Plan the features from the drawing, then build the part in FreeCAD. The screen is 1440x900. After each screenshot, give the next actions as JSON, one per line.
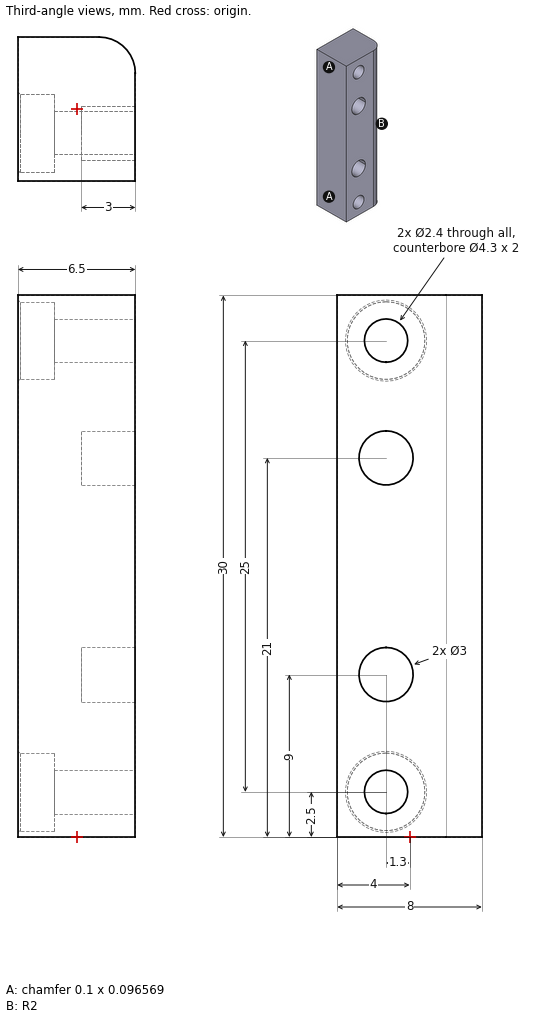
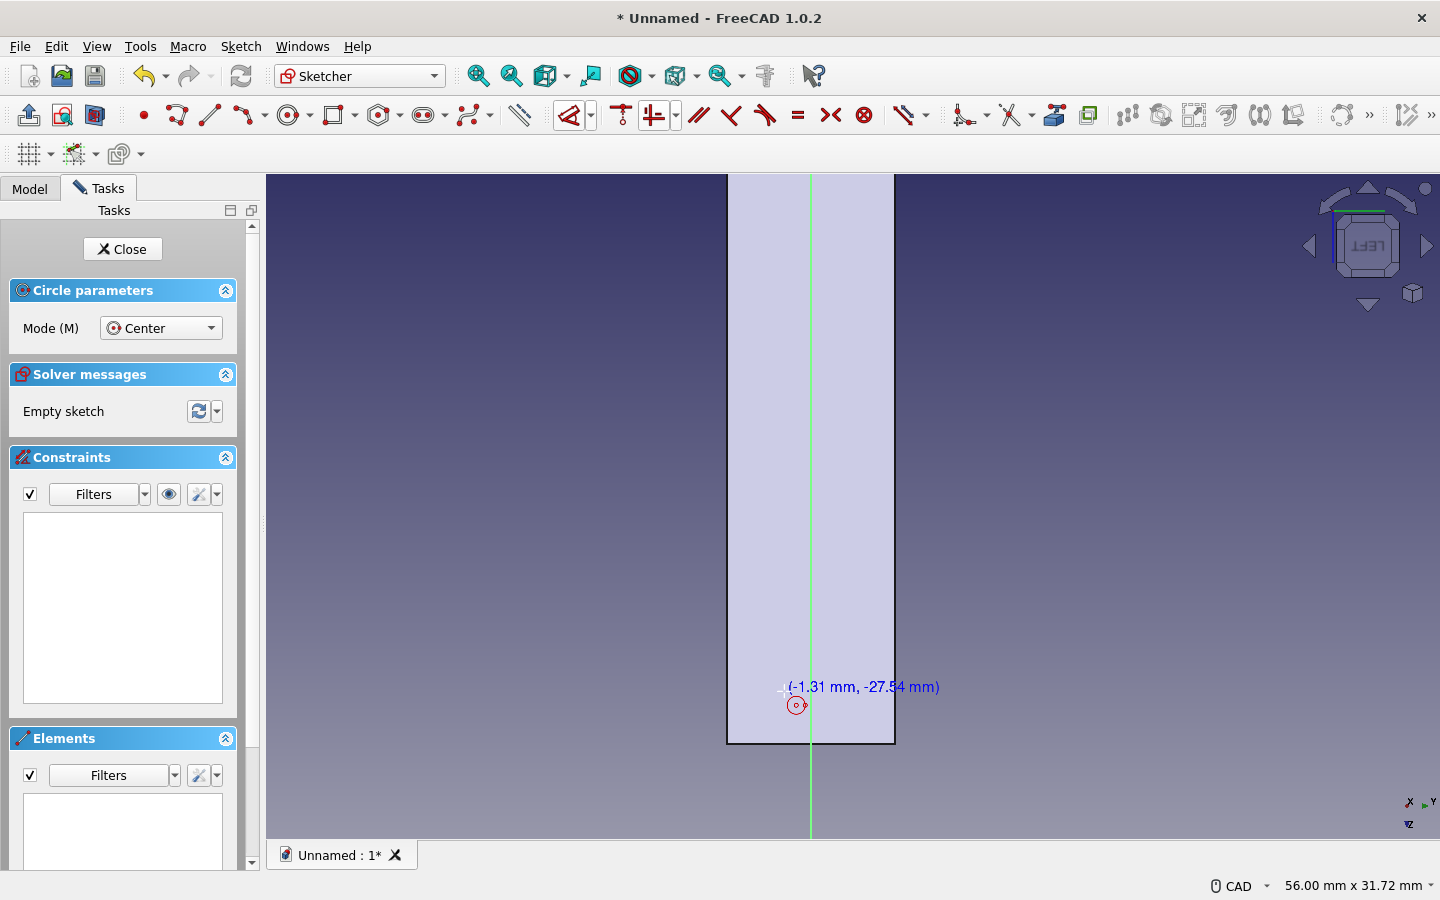
{"action": "left_click", "coordinate": [784, 691]}
{"action": "mouse_move", "coordinate": [766, 673]}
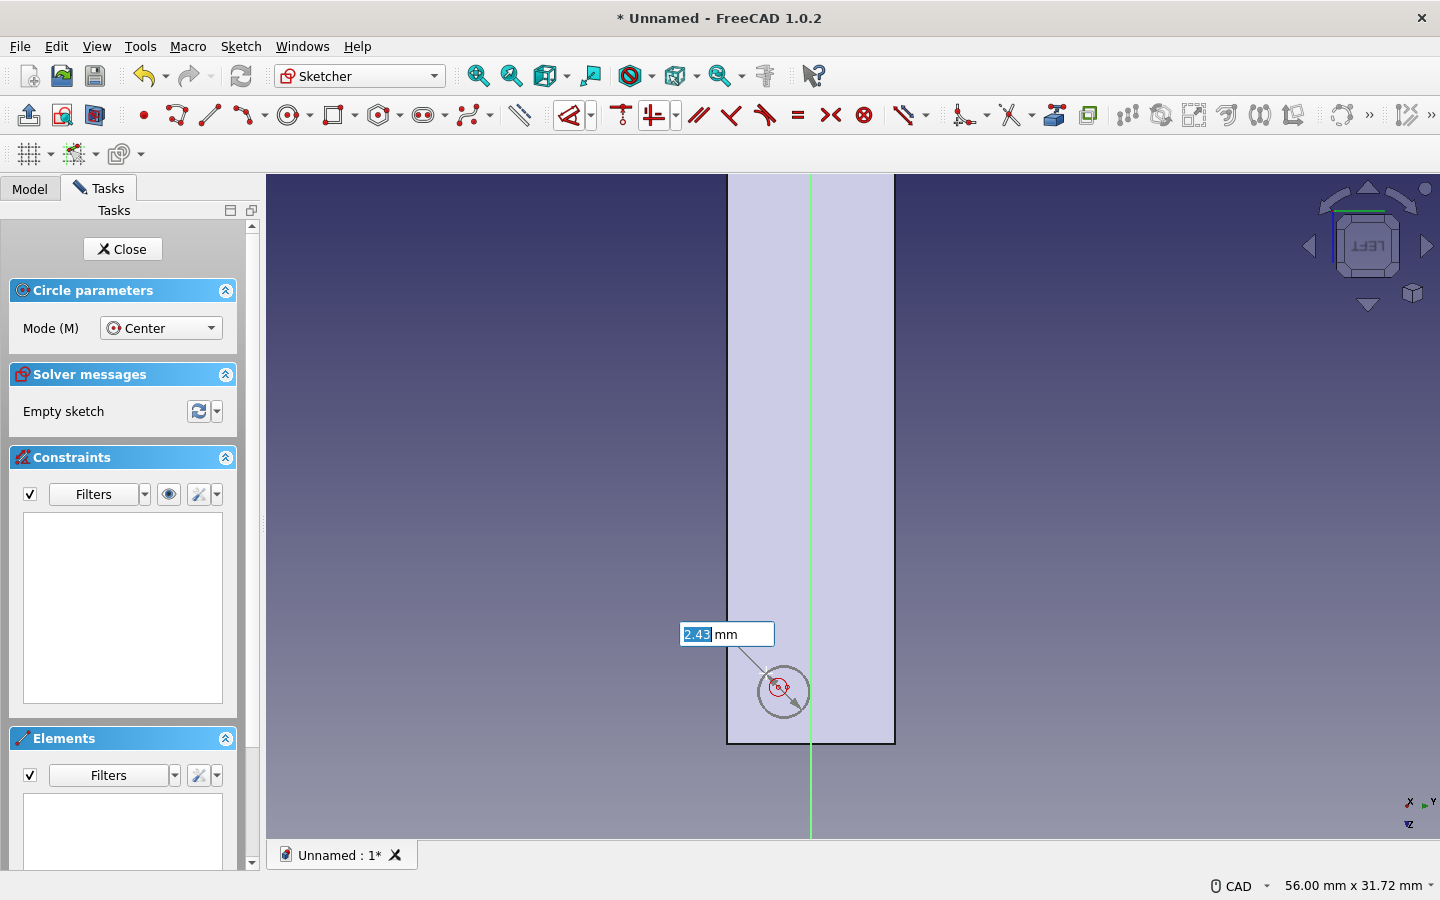
{"action": "type", "text": "2.4"}
{"action": "key", "text": "Return"}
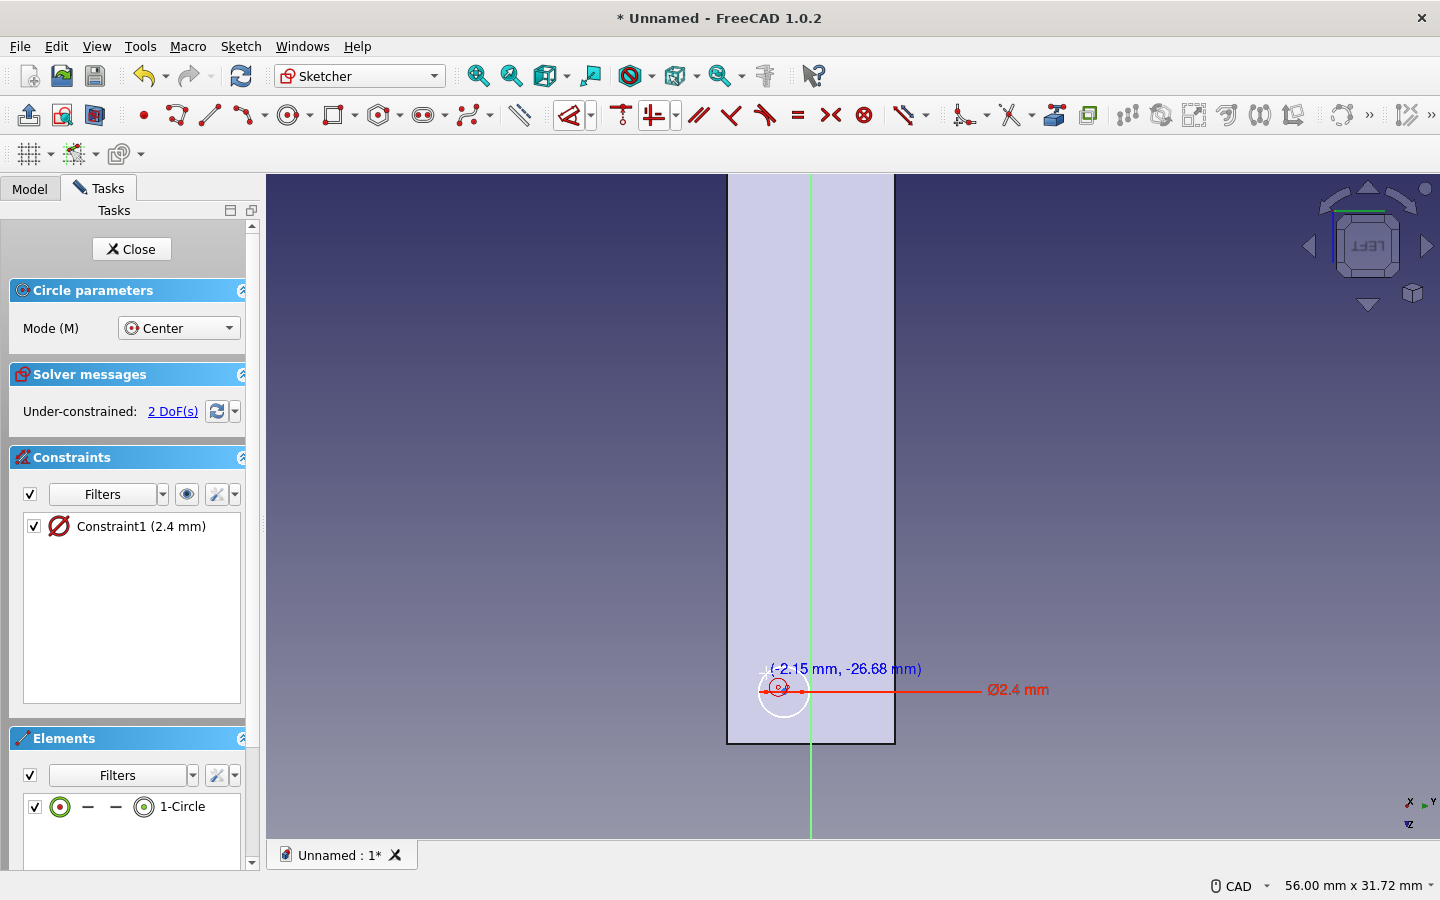
{"action": "scroll", "coordinate": [784, 691], "scroll_direction": "down", "scroll_amount": 2}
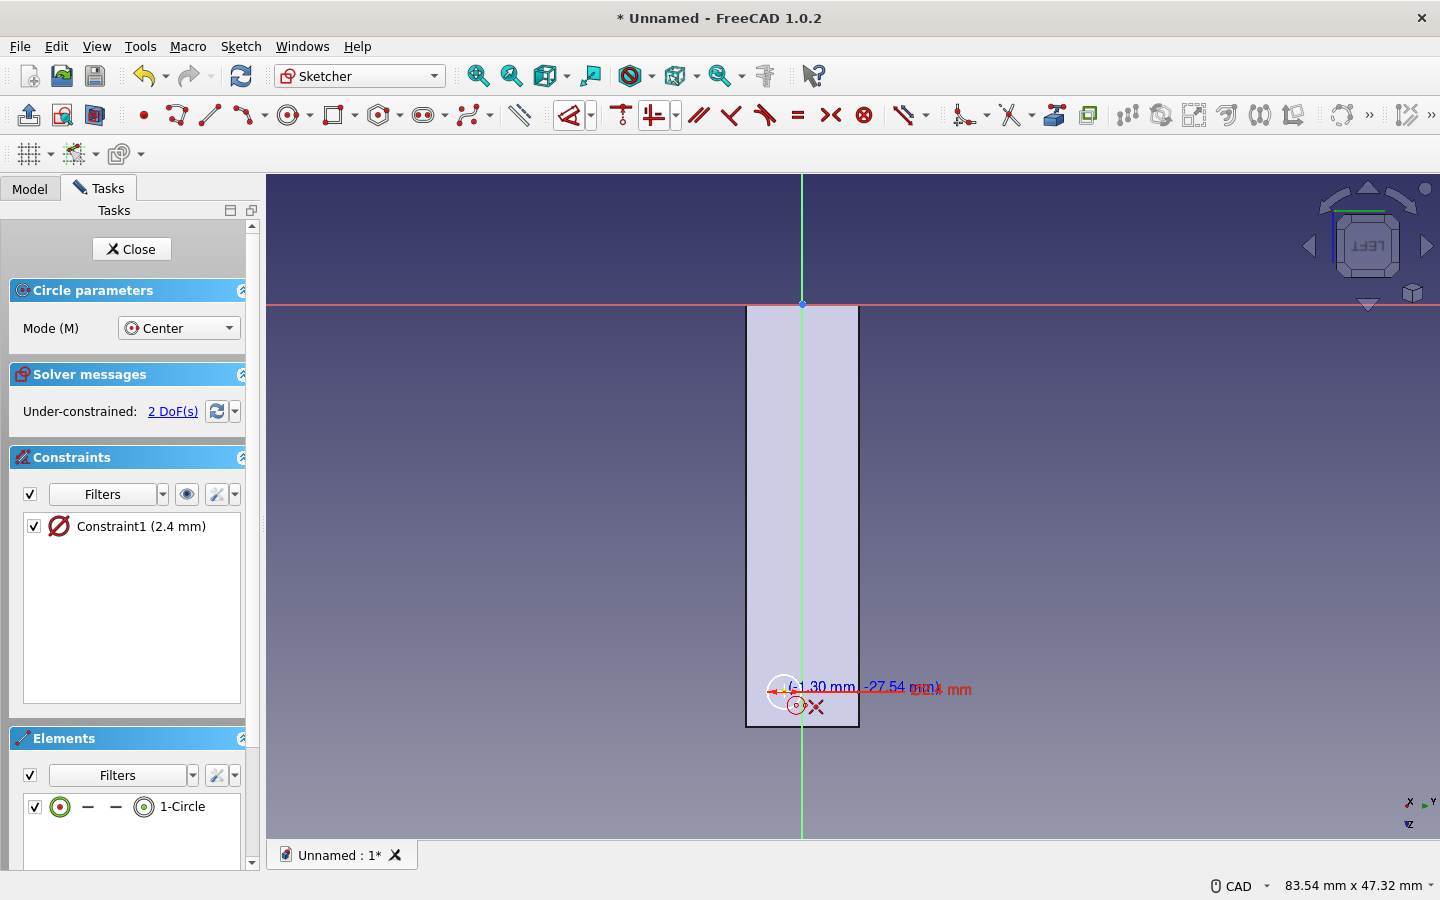
{"action": "scroll", "coordinate": [784, 340], "scroll_direction": "up", "scroll_amount": 2}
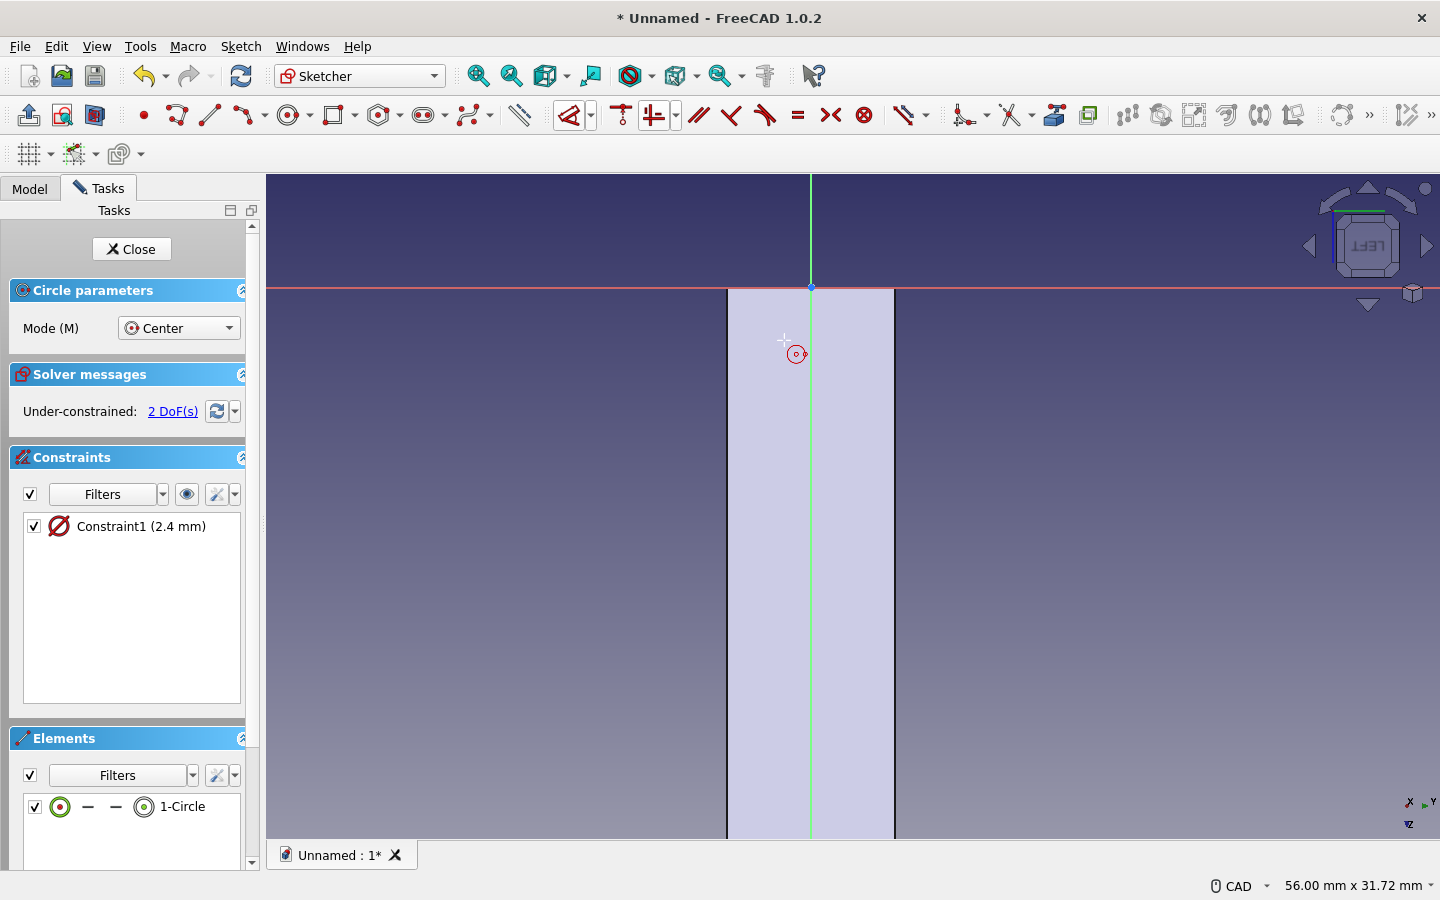
{"action": "left_click", "coordinate": [784, 340]}
{"action": "mouse_move", "coordinate": [766, 322]}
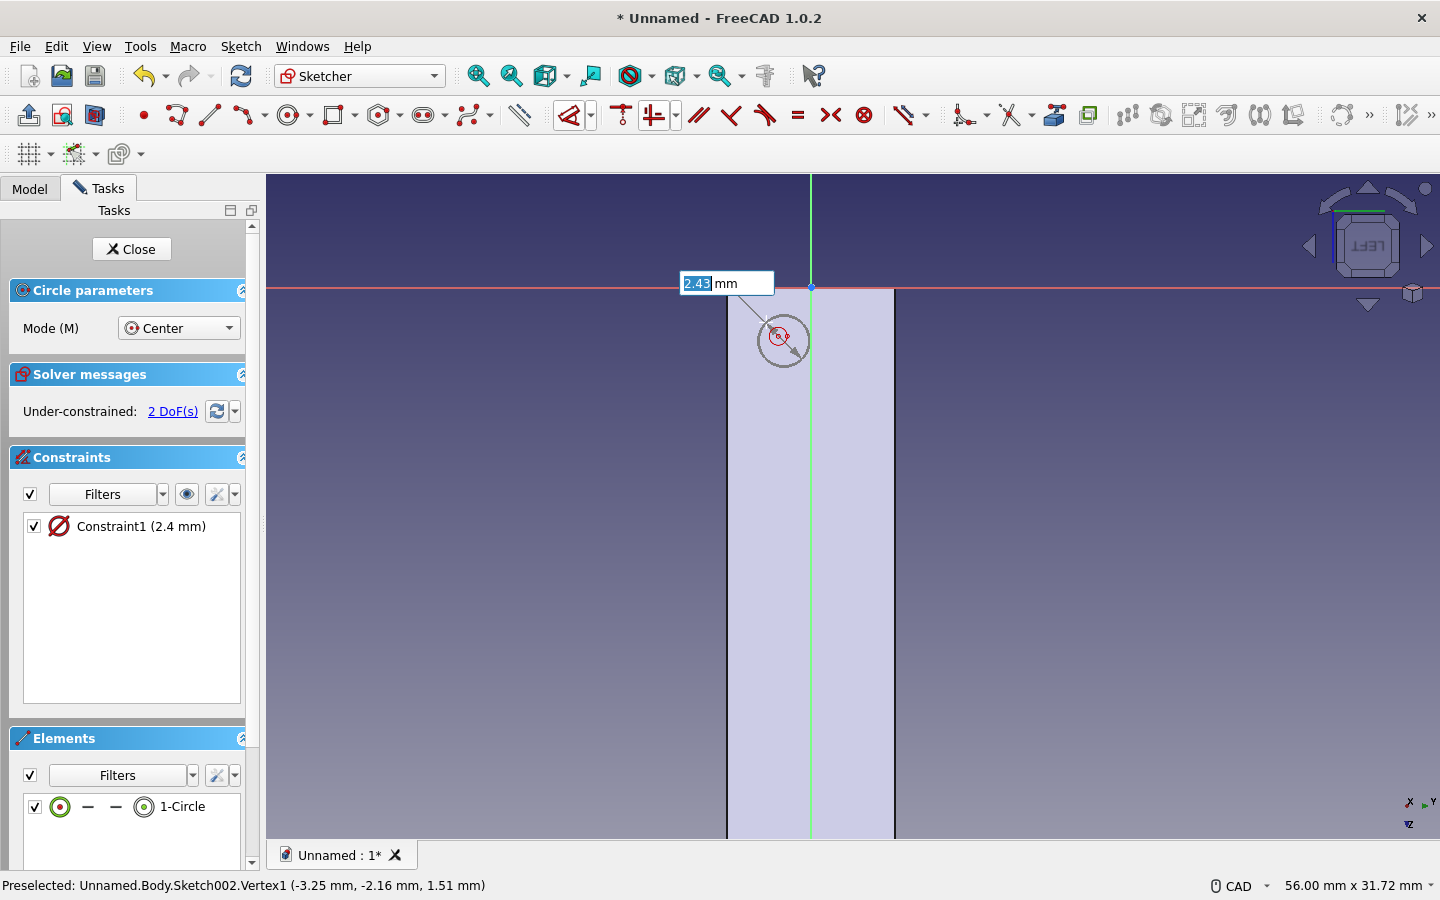
{"action": "type", "text": "2.4"}
{"action": "key", "text": "Return"}
{"action": "key", "text": "Escape"}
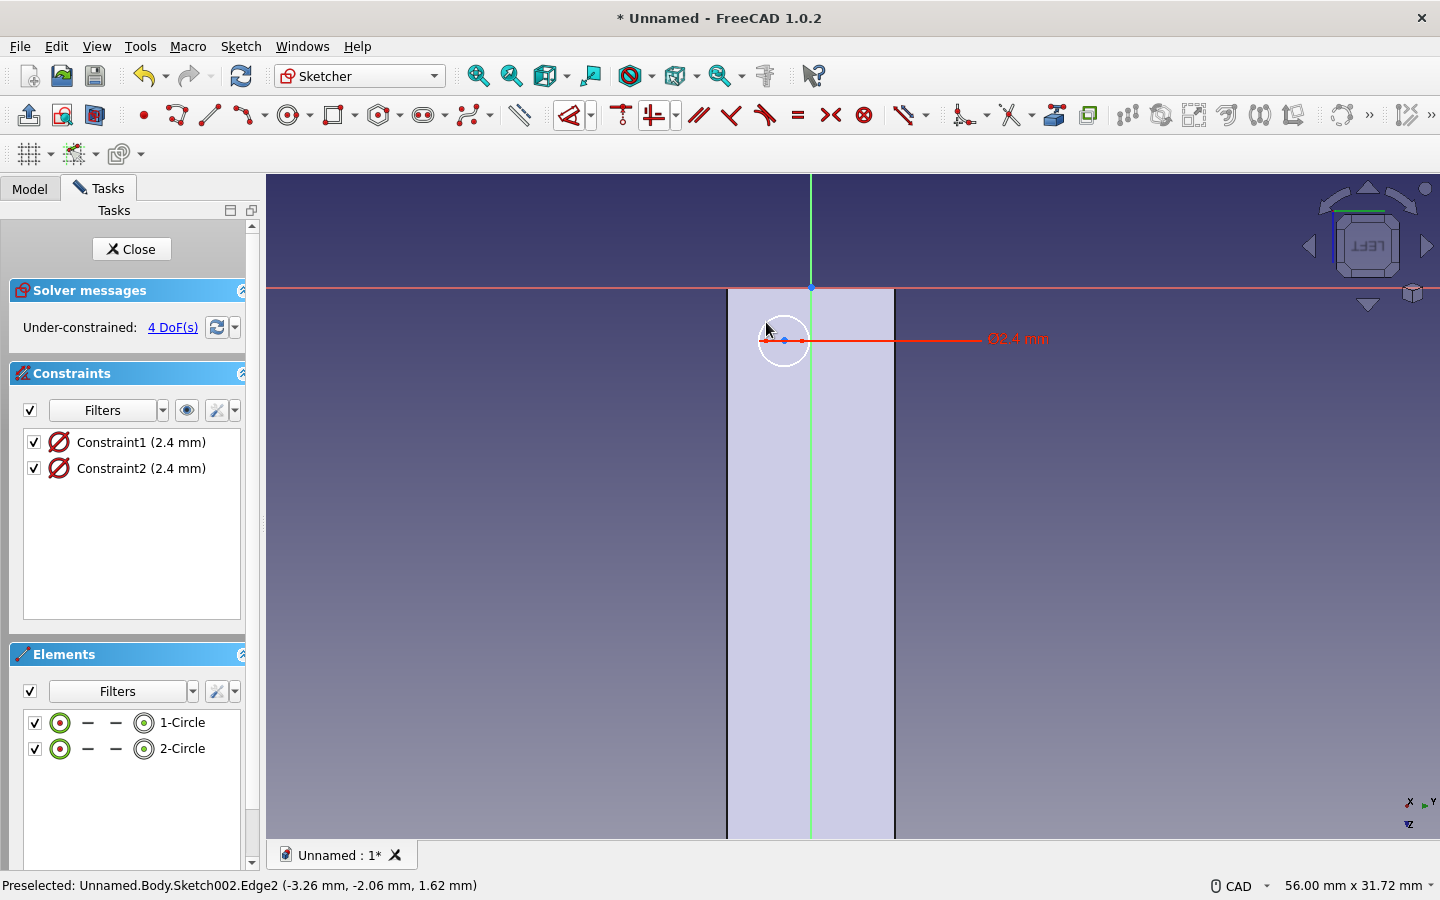
{"action": "scroll", "coordinate": [784, 340], "scroll_direction": "down", "scroll_amount": 2}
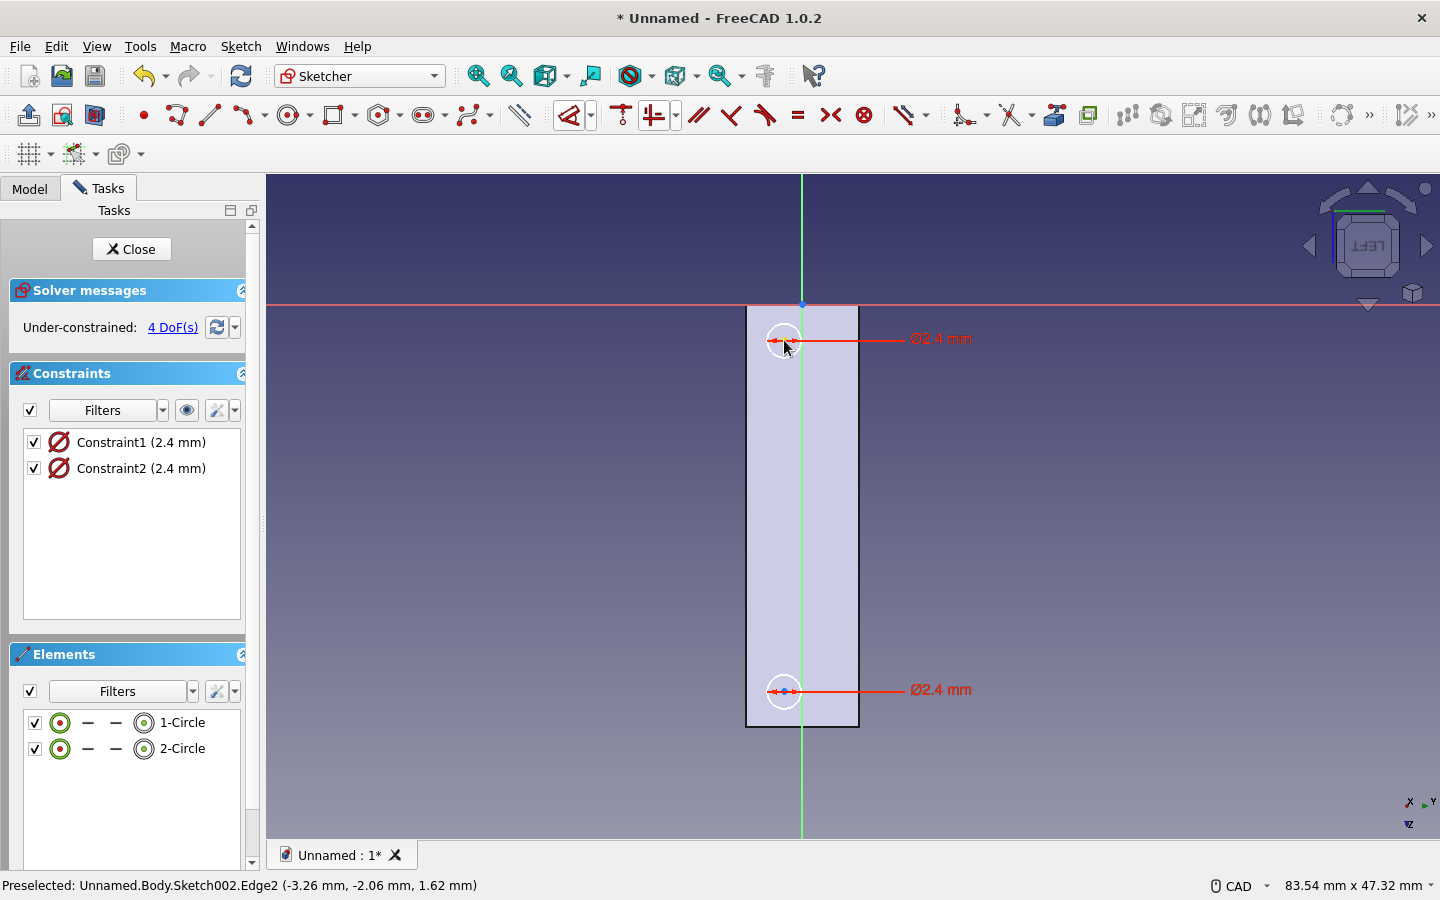
{"action": "left_click", "coordinate": [784, 692]}